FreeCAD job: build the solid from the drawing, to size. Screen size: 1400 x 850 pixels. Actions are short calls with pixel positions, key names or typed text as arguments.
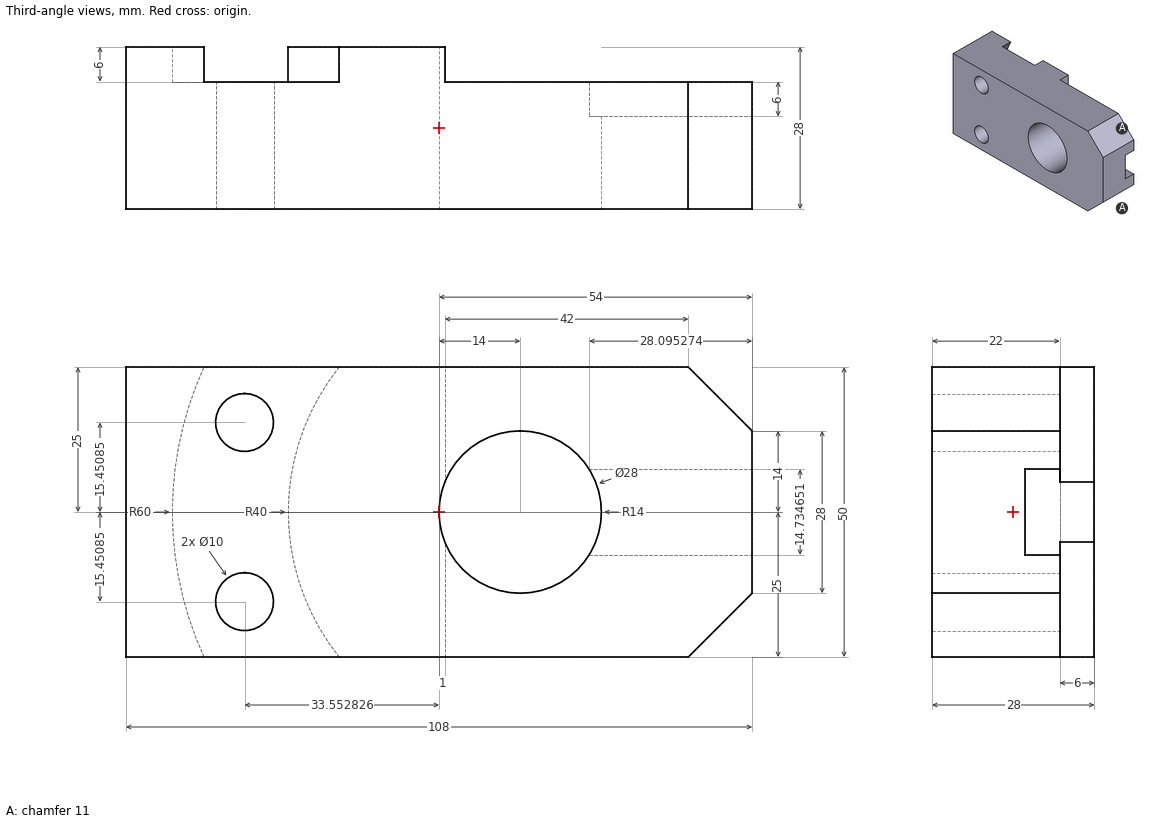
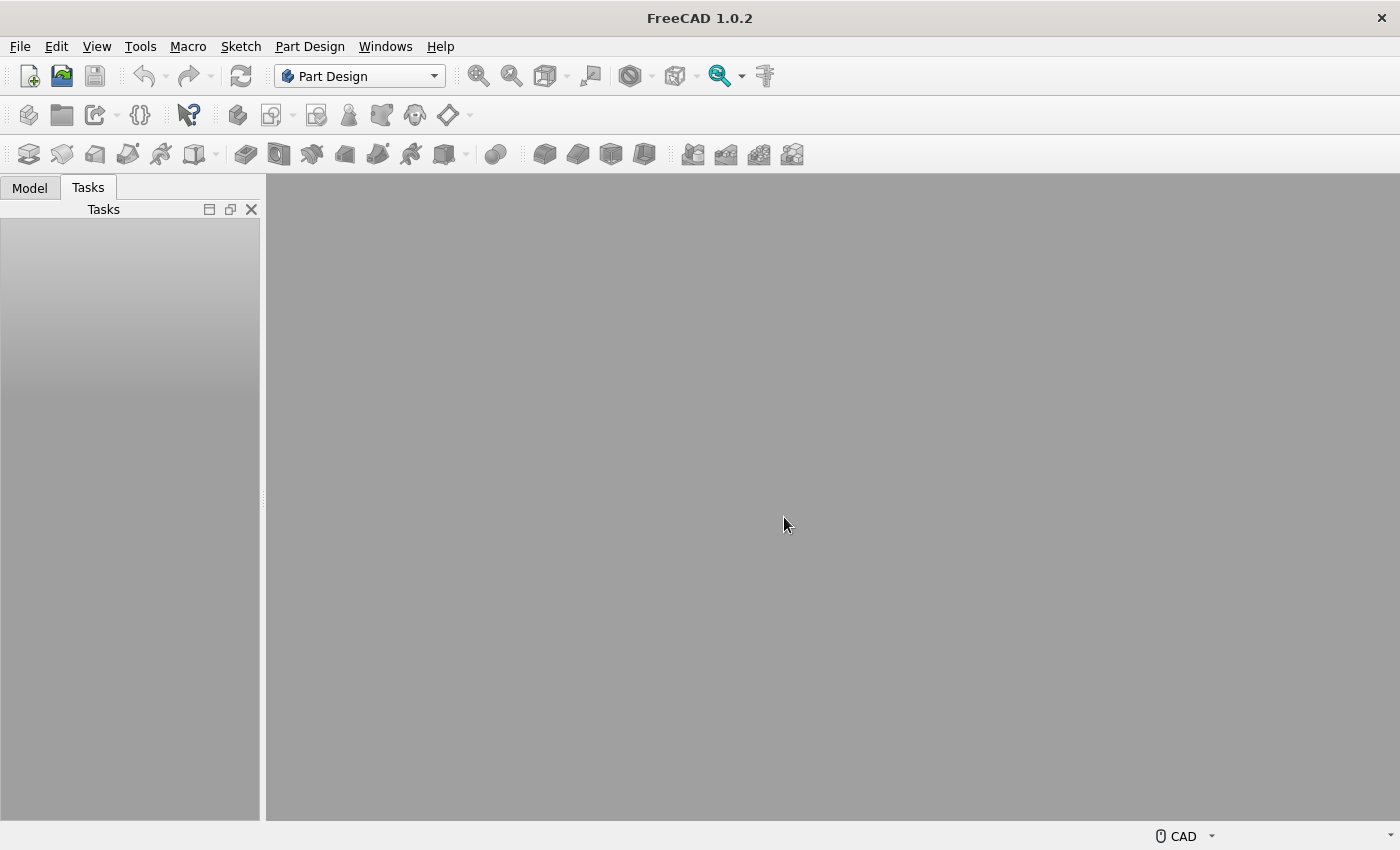
key(ctrl+n)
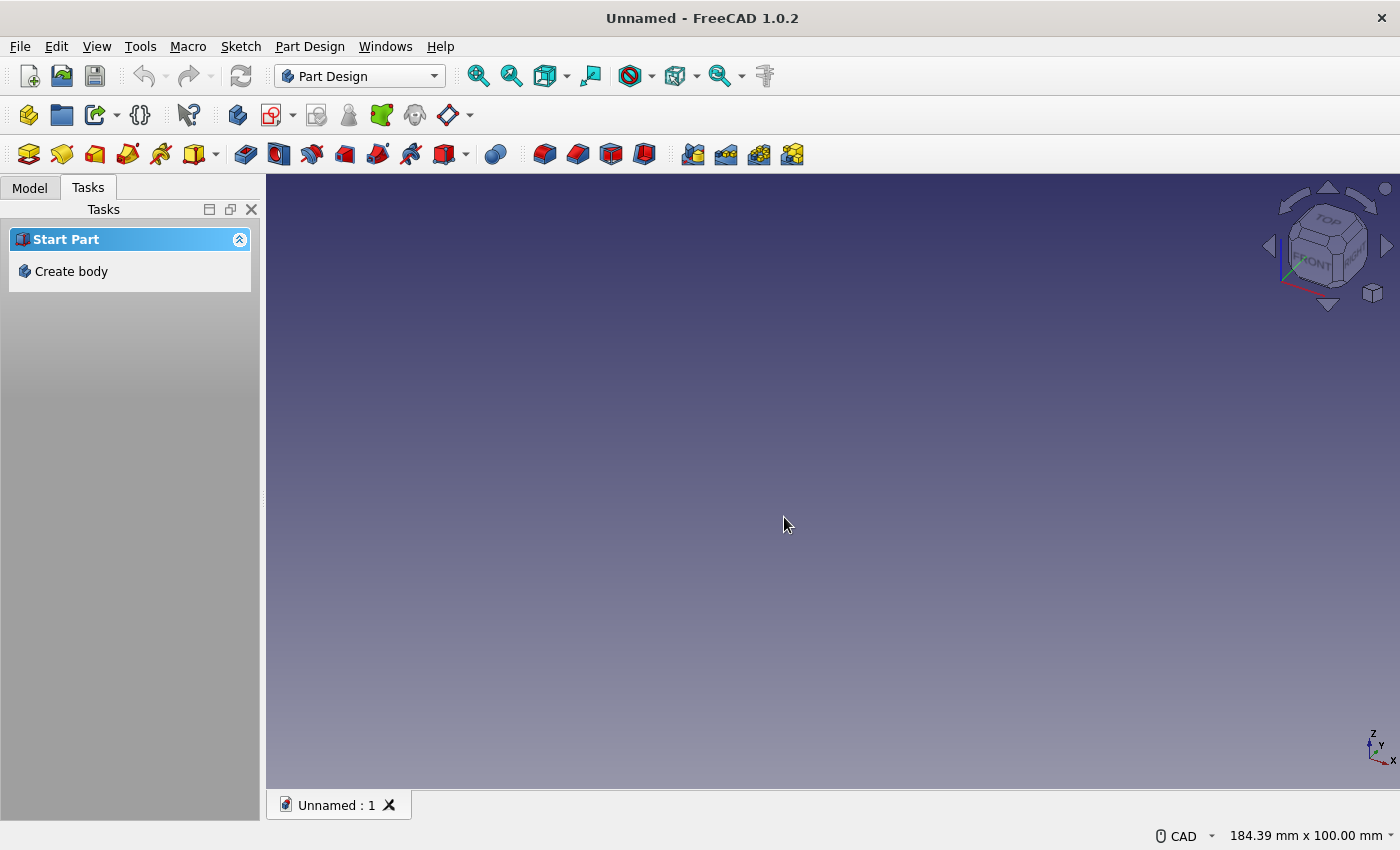
click(270, 116)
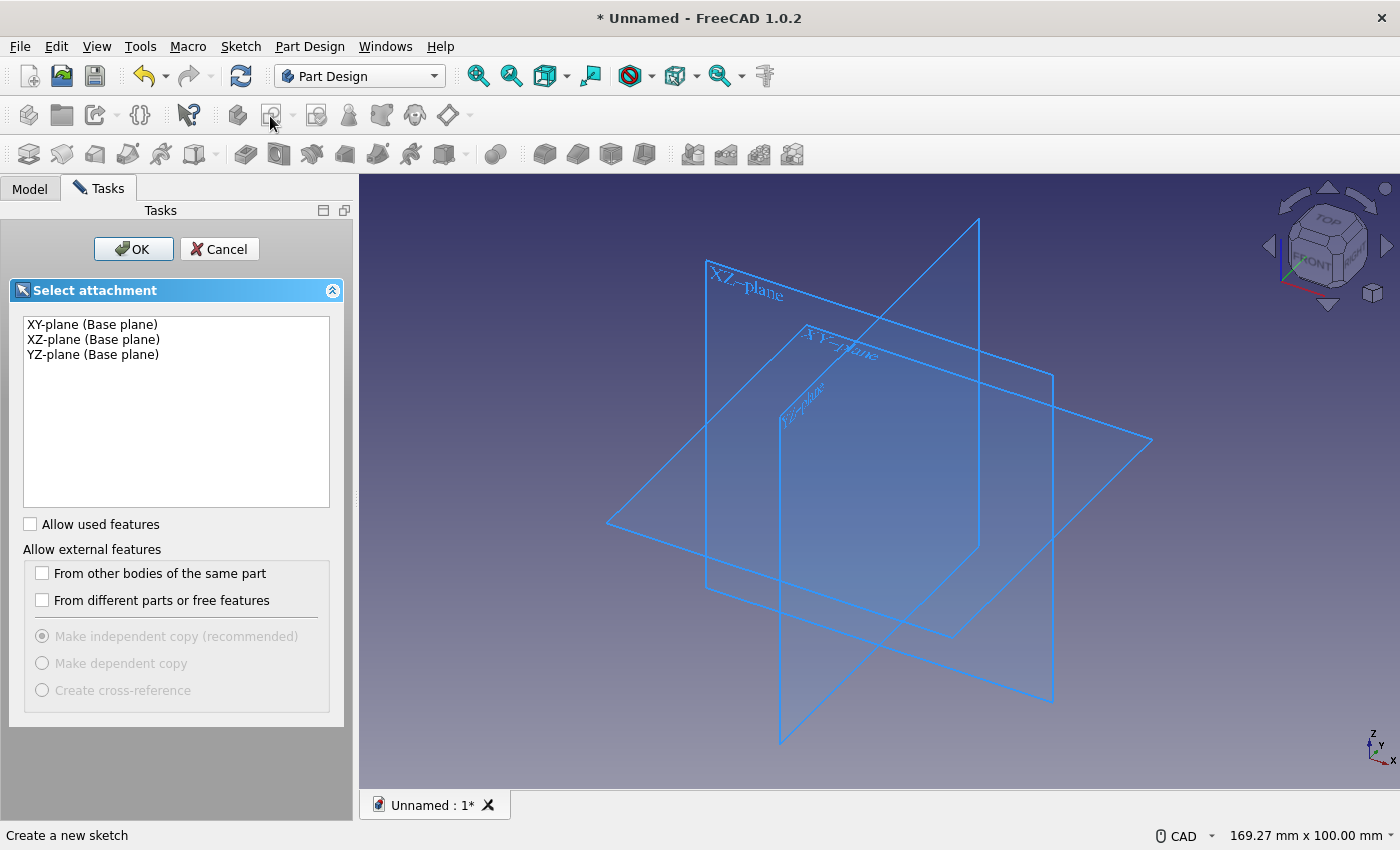
click(84, 340)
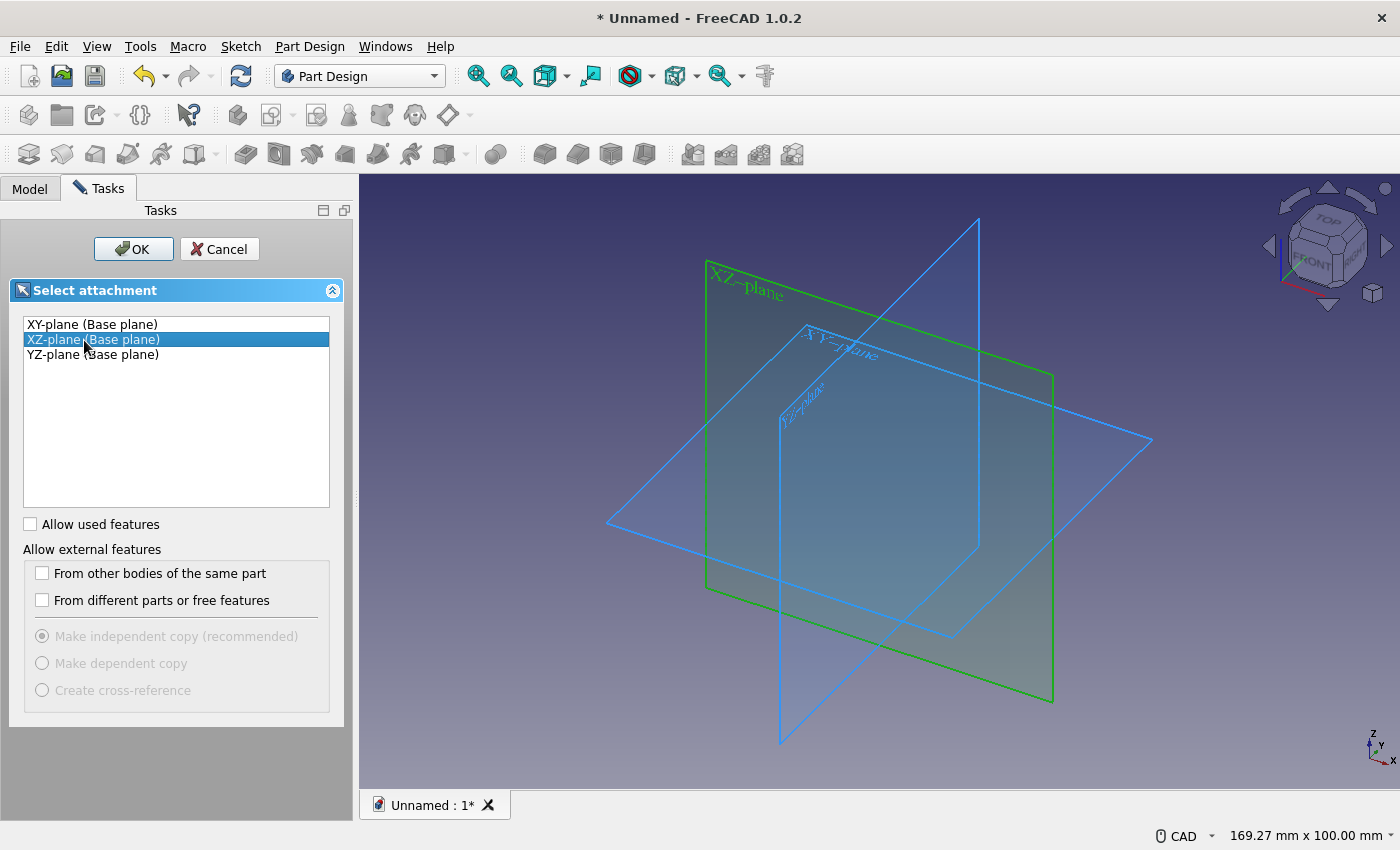
click(134, 249)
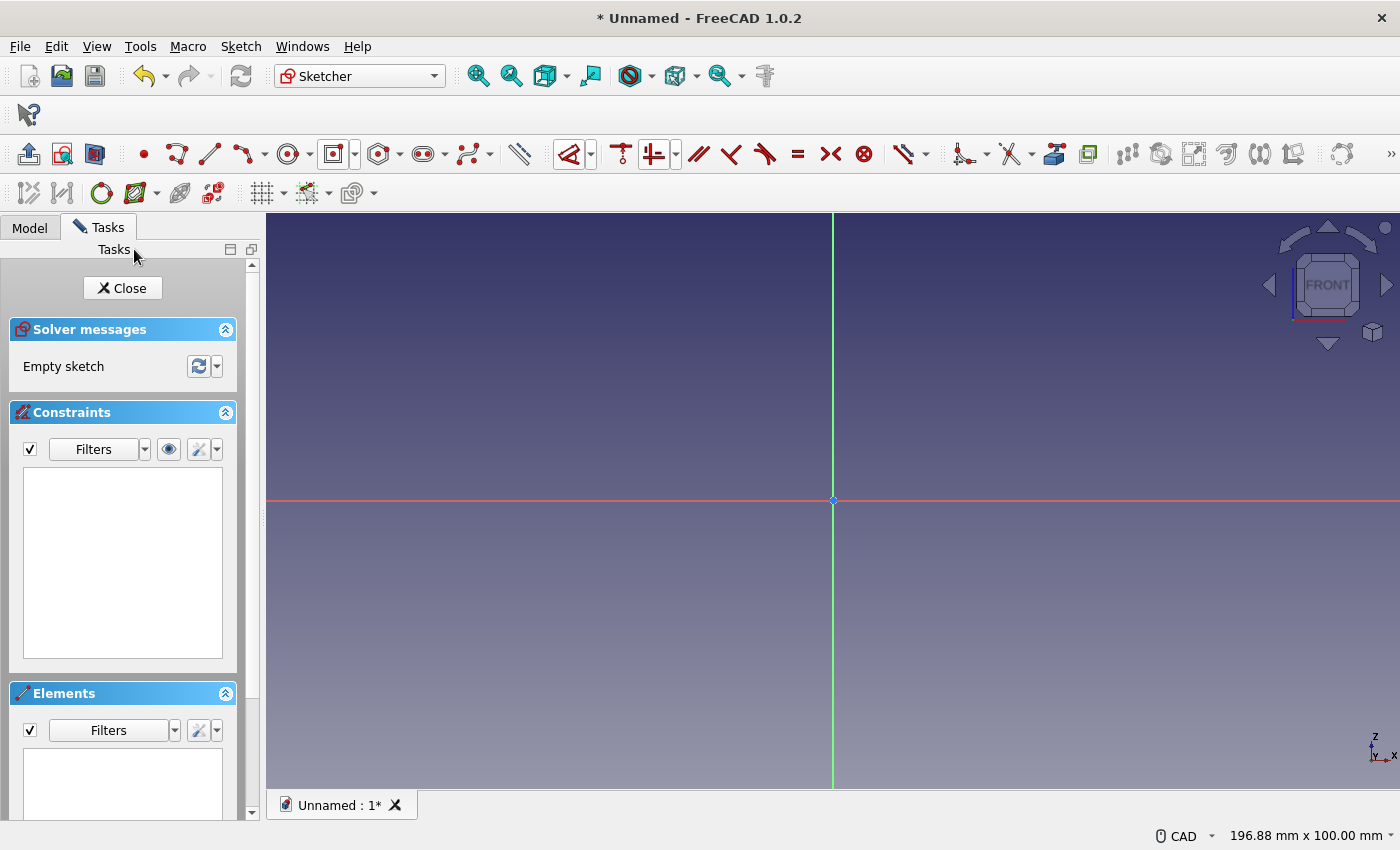
click(332, 154)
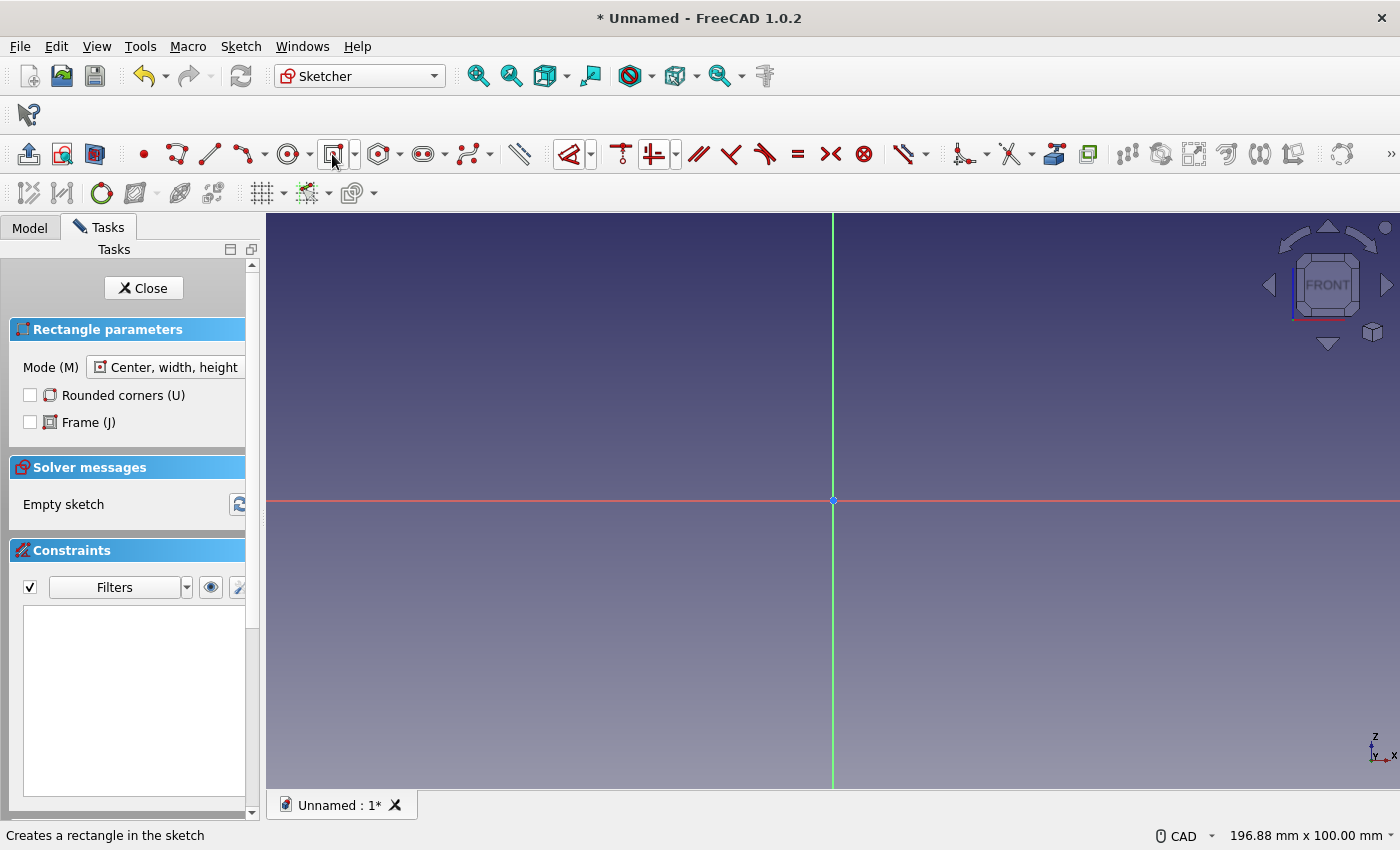
click(833, 501)
move(1144, 357)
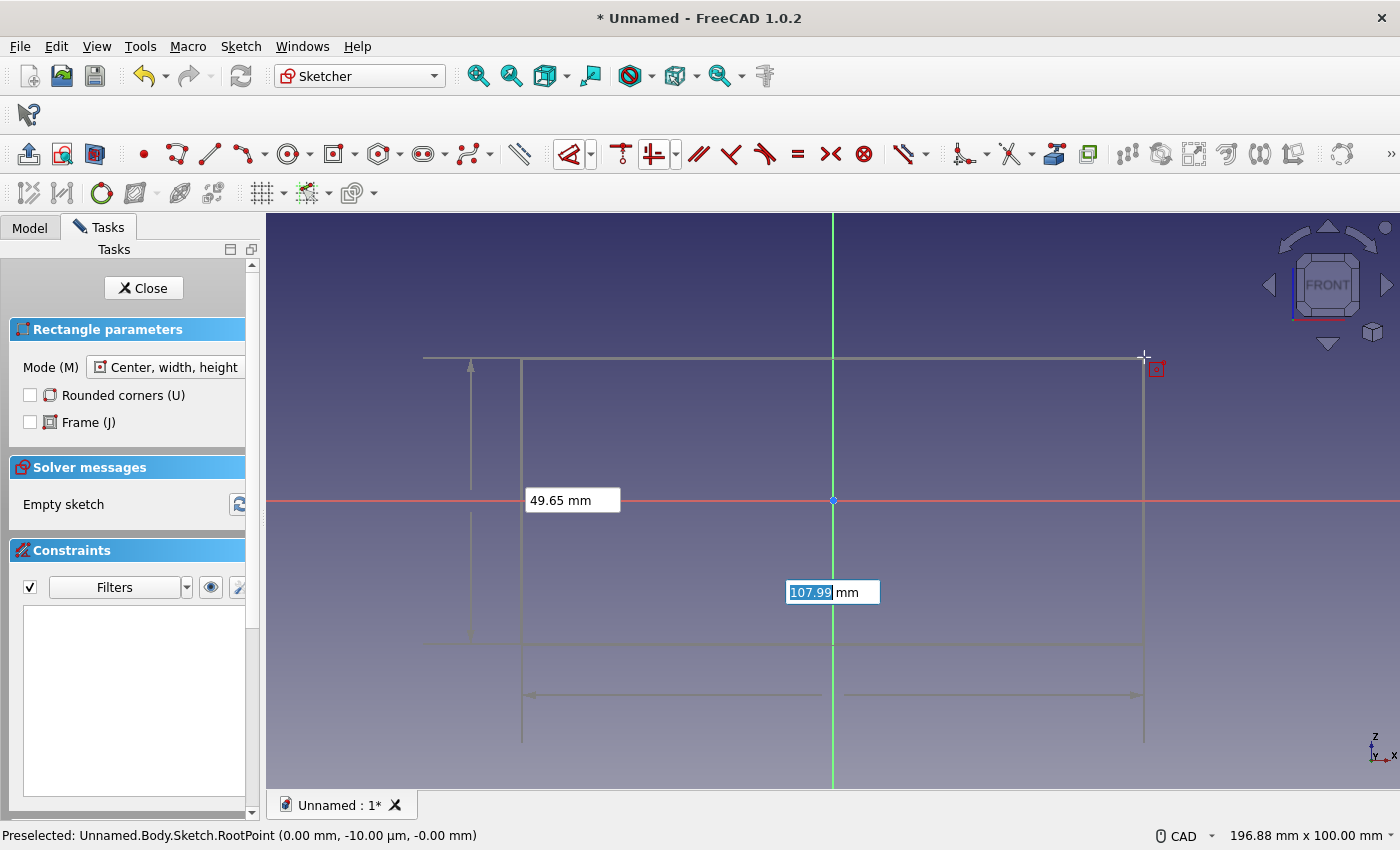
text(108)
key(Tab)
text(50)
key(Return)
key(Escape)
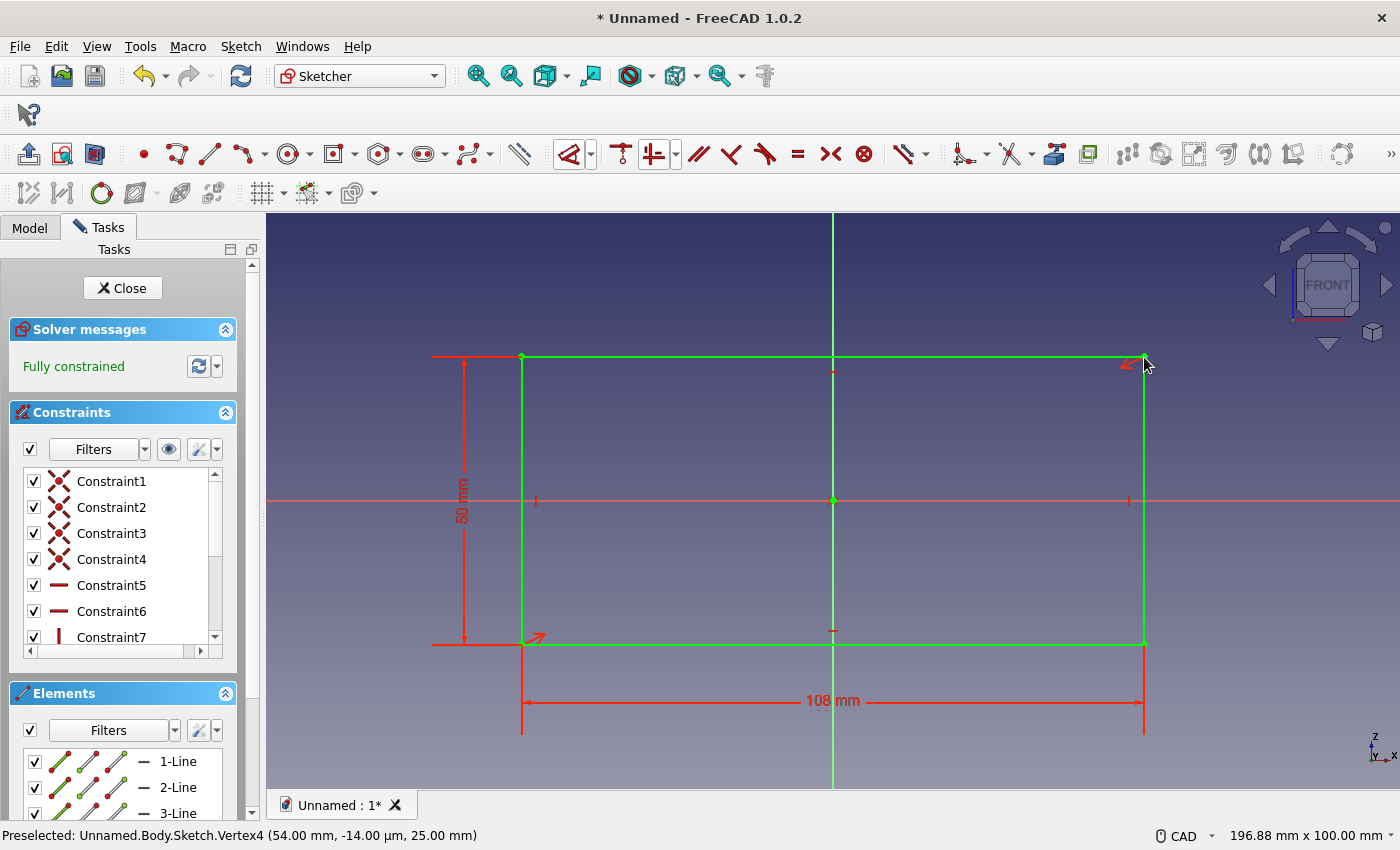
click(123, 288)